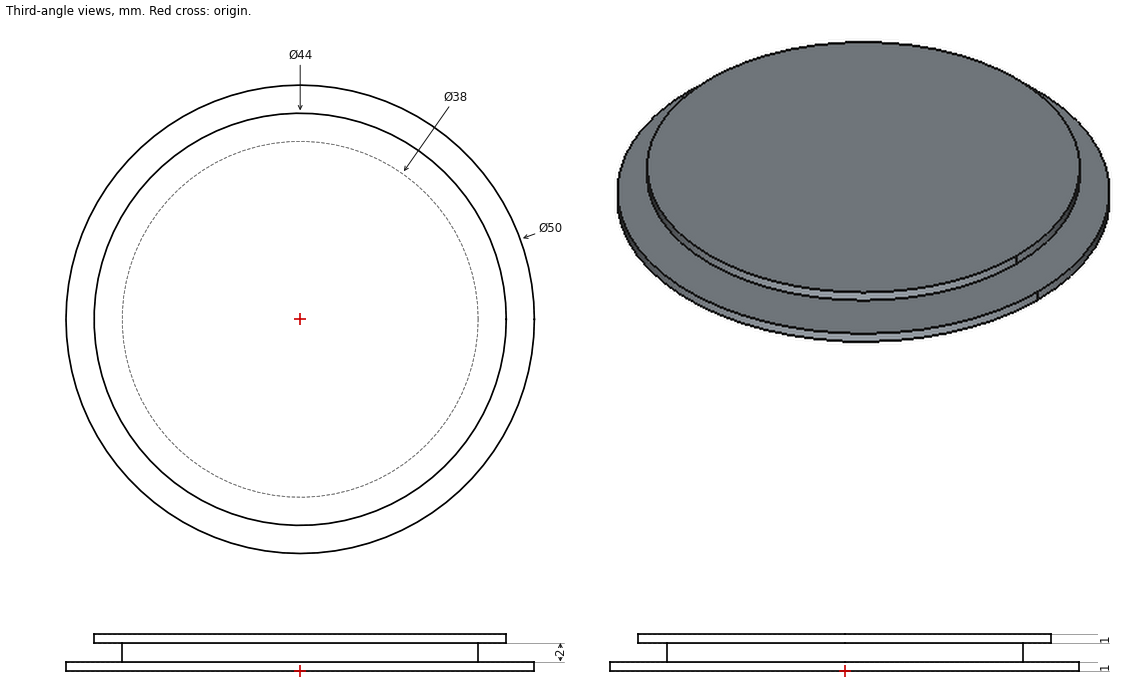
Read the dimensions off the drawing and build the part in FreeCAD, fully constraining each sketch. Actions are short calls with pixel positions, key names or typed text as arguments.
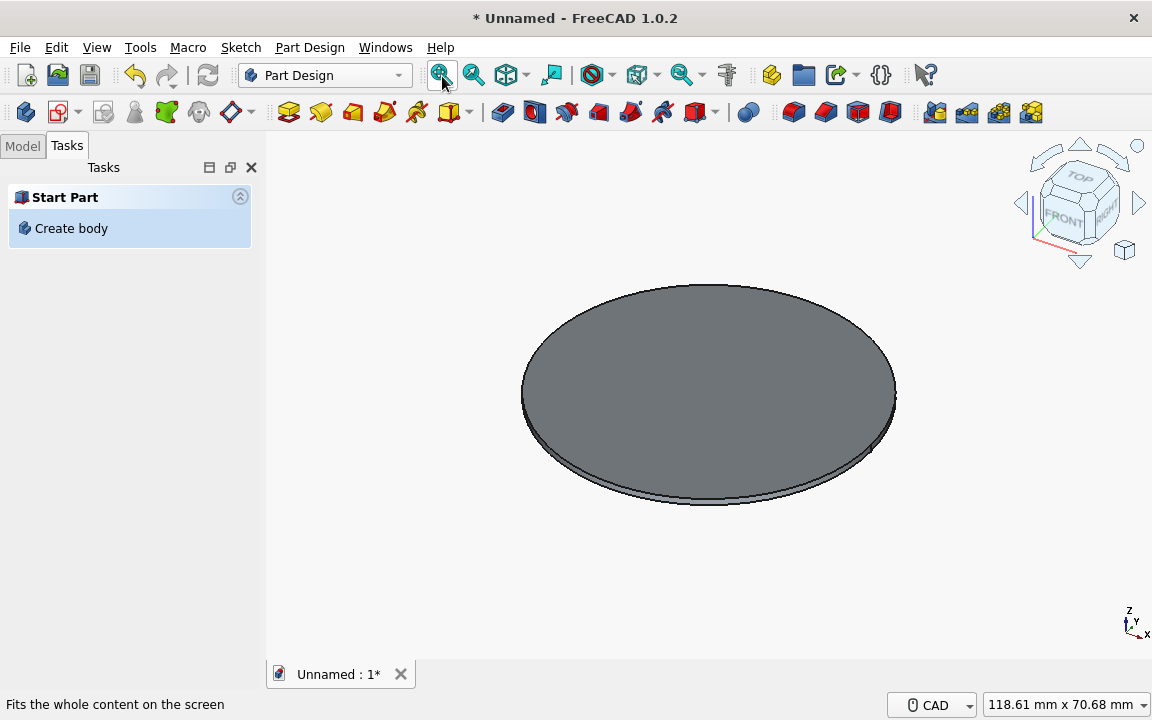
click(709, 391)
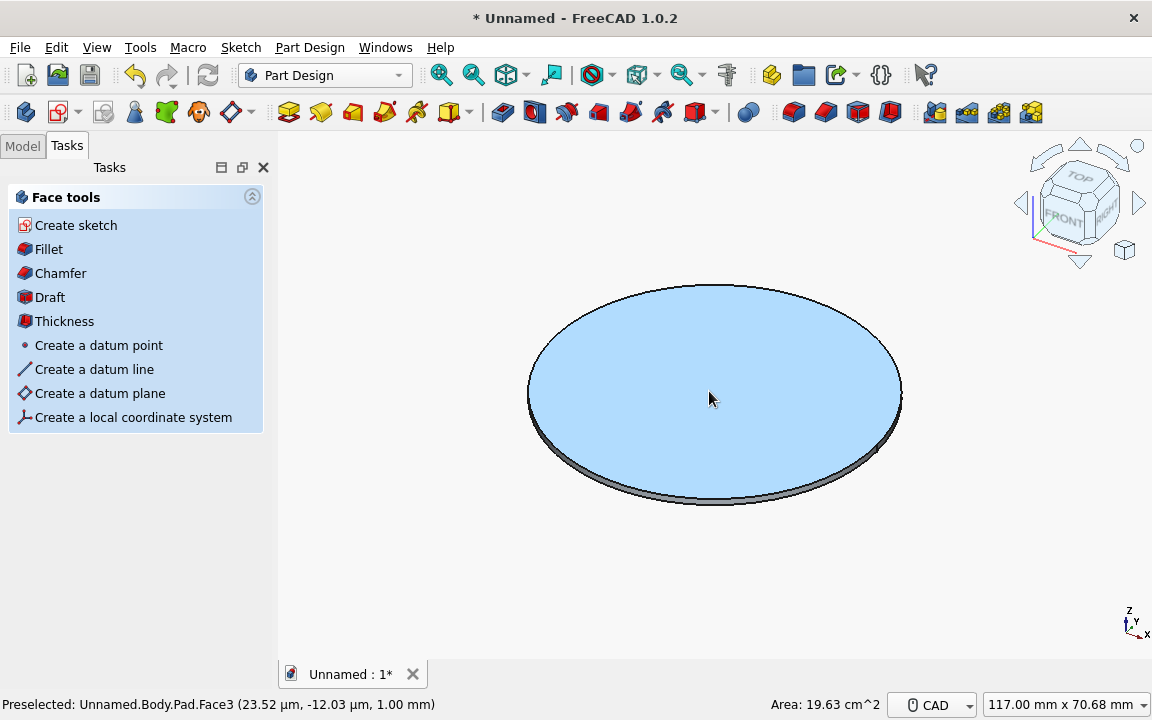
click(58, 112)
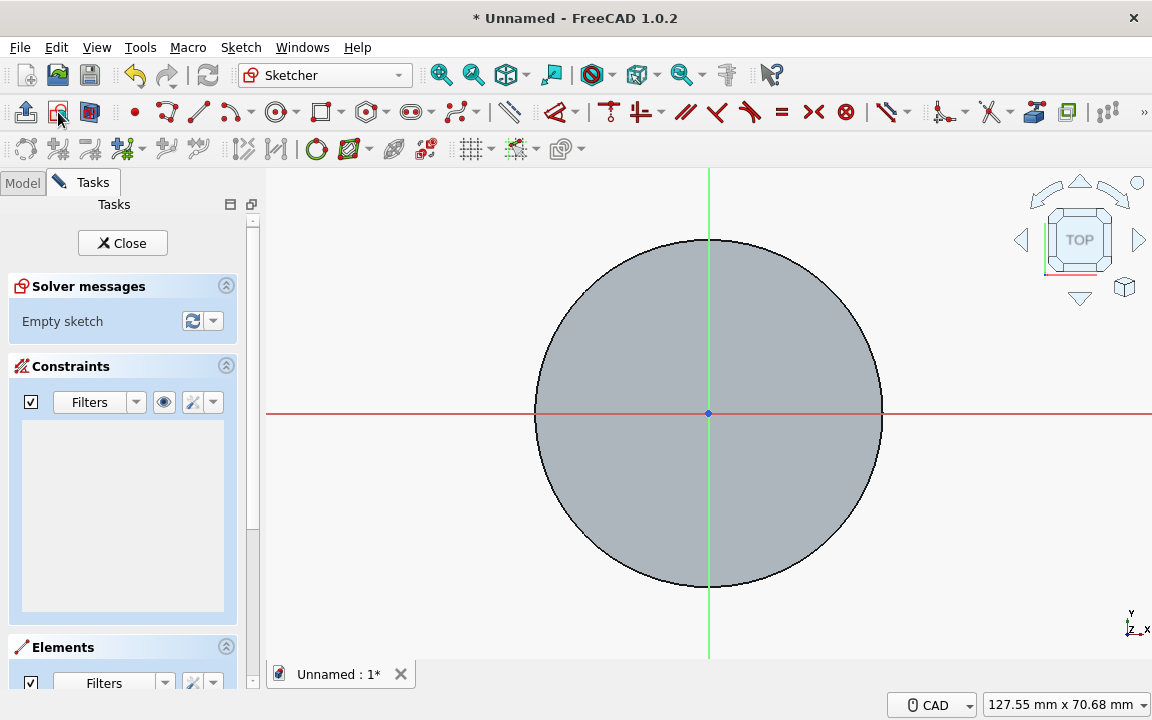
click(276, 112)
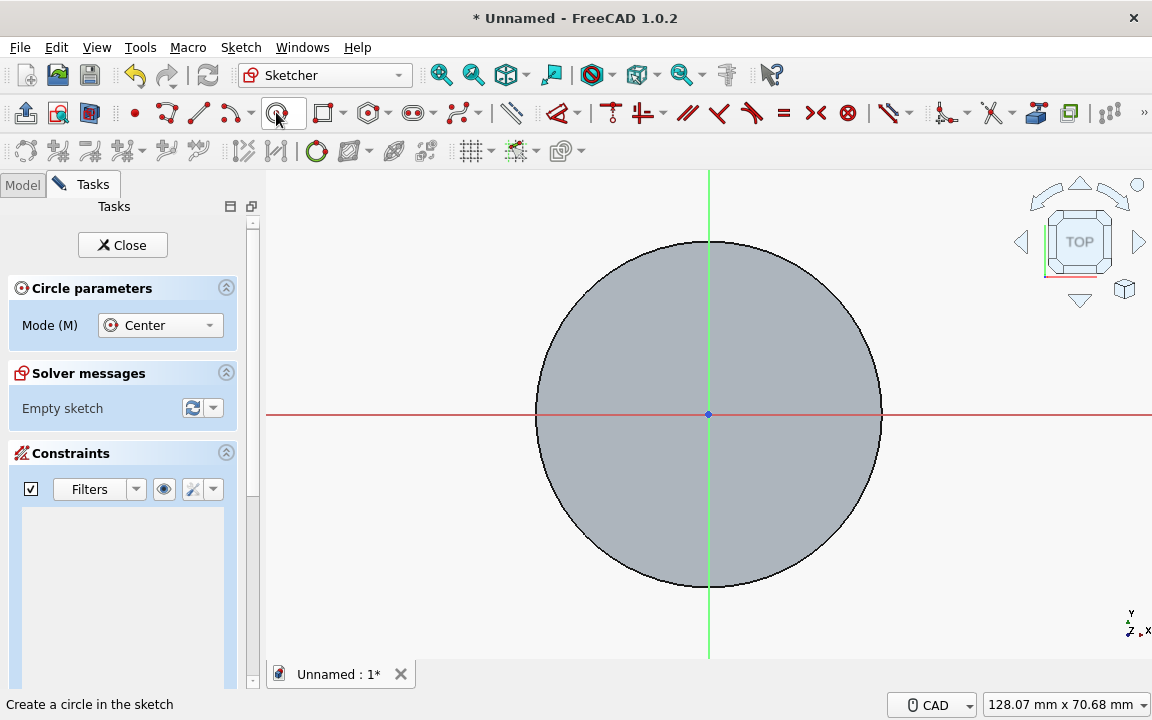
click(709, 414)
move(802, 322)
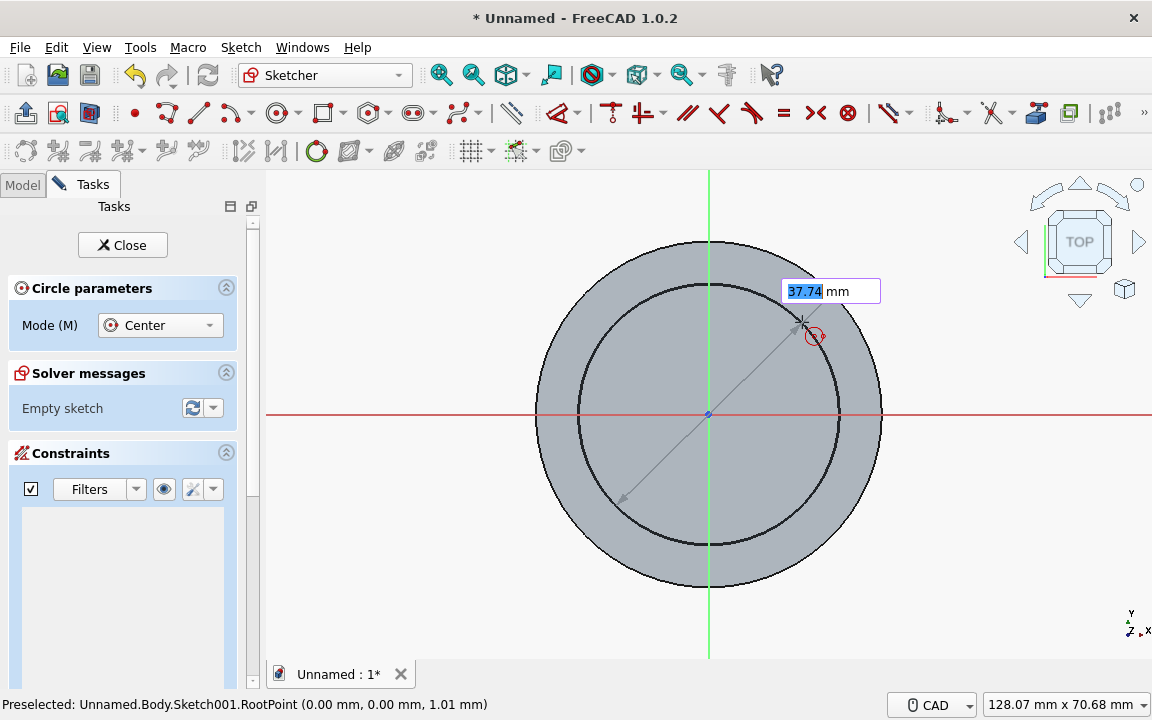
text(38)
key(Return)
key(Escape)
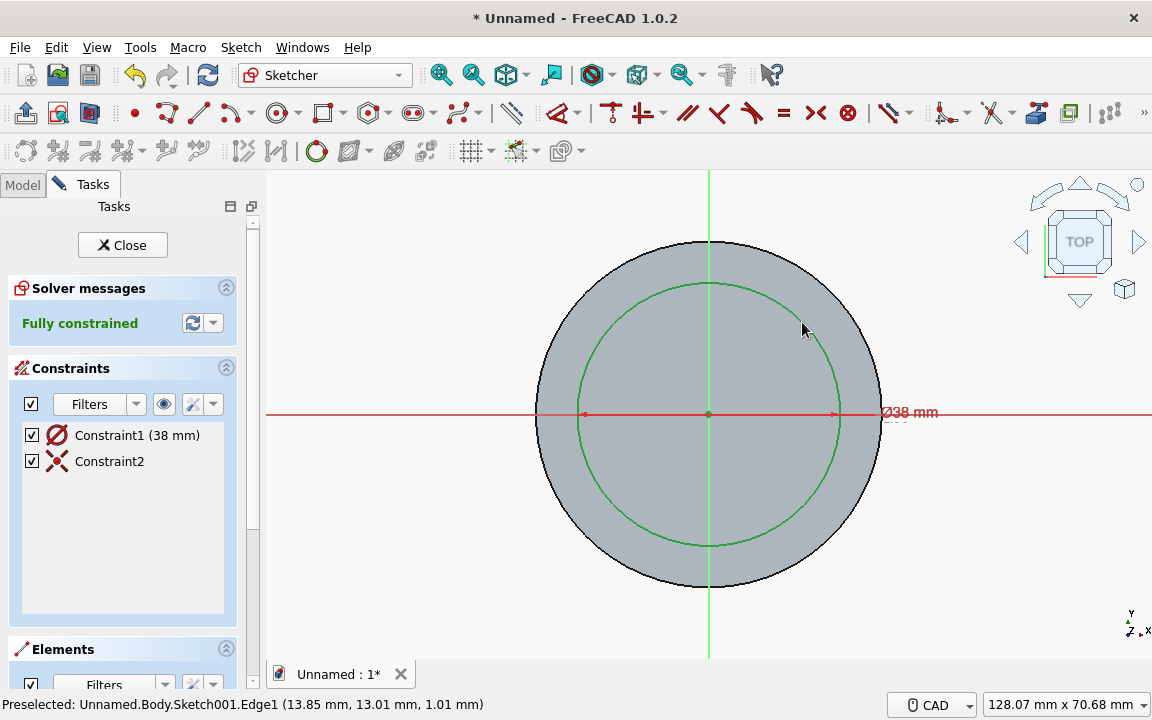
click(123, 245)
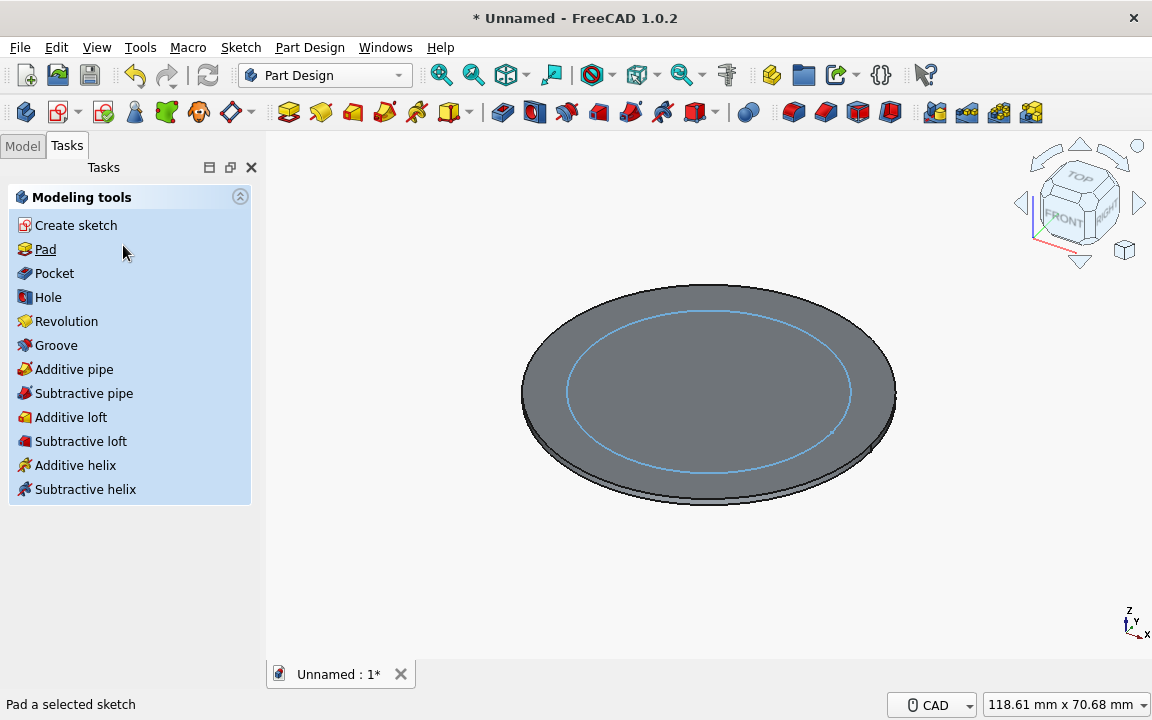
click(290, 112)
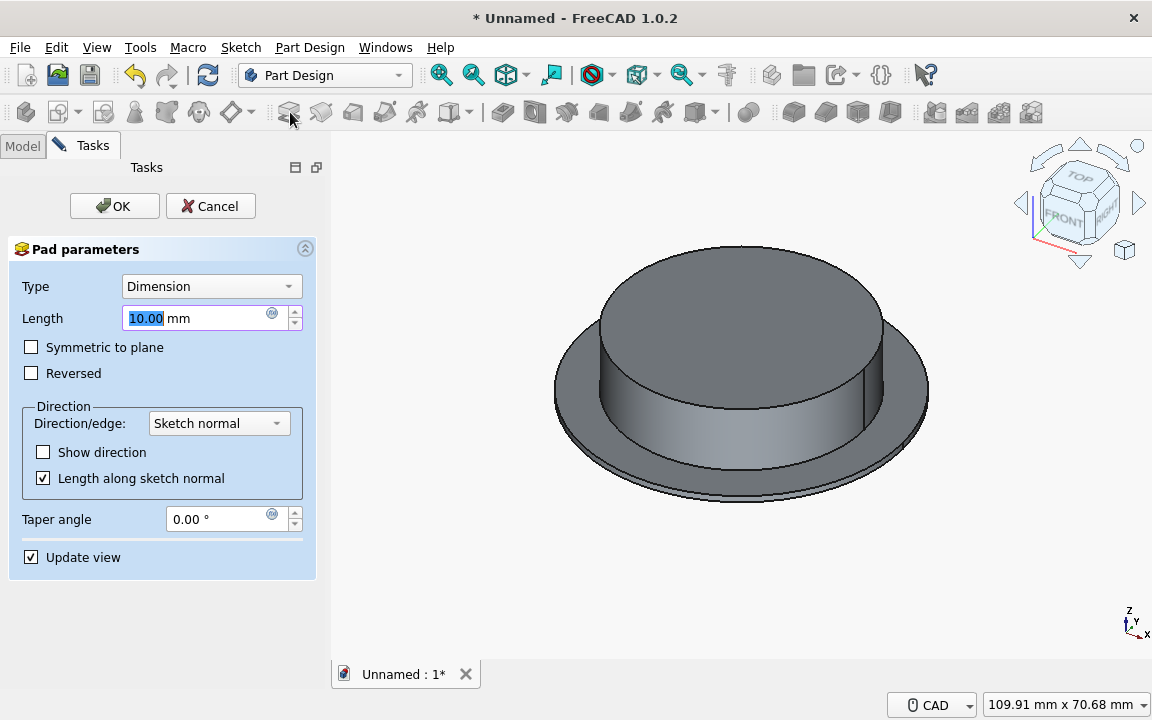
text(2)
key(Tab)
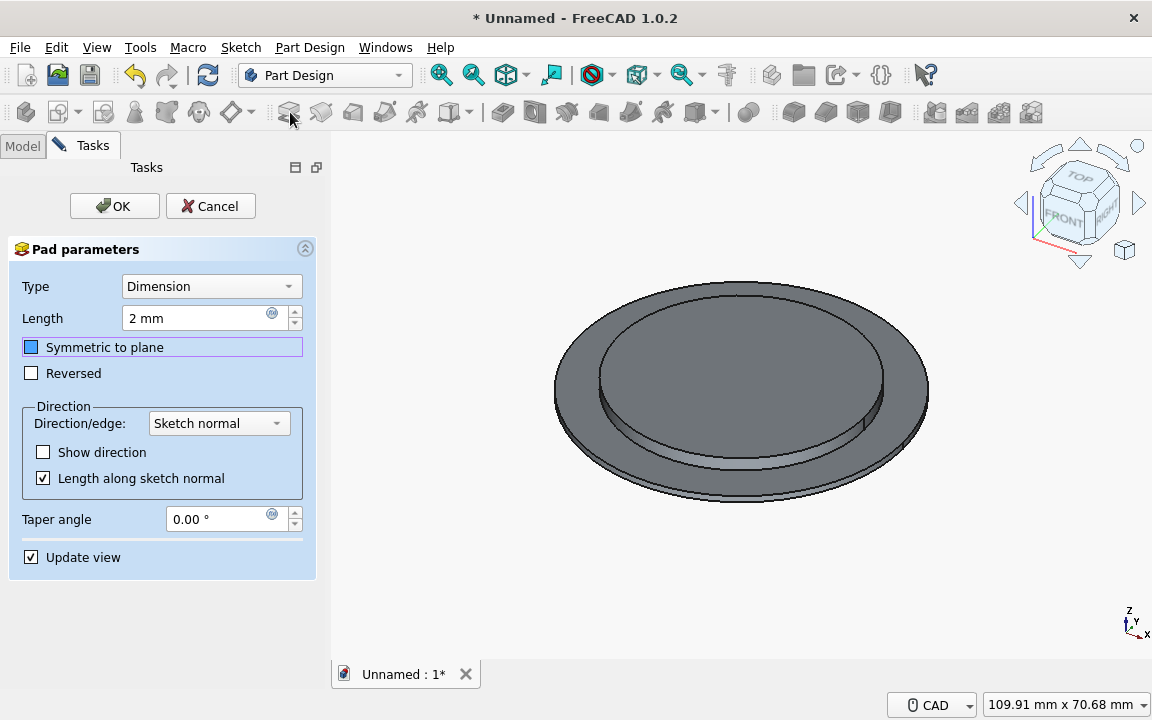
click(115, 206)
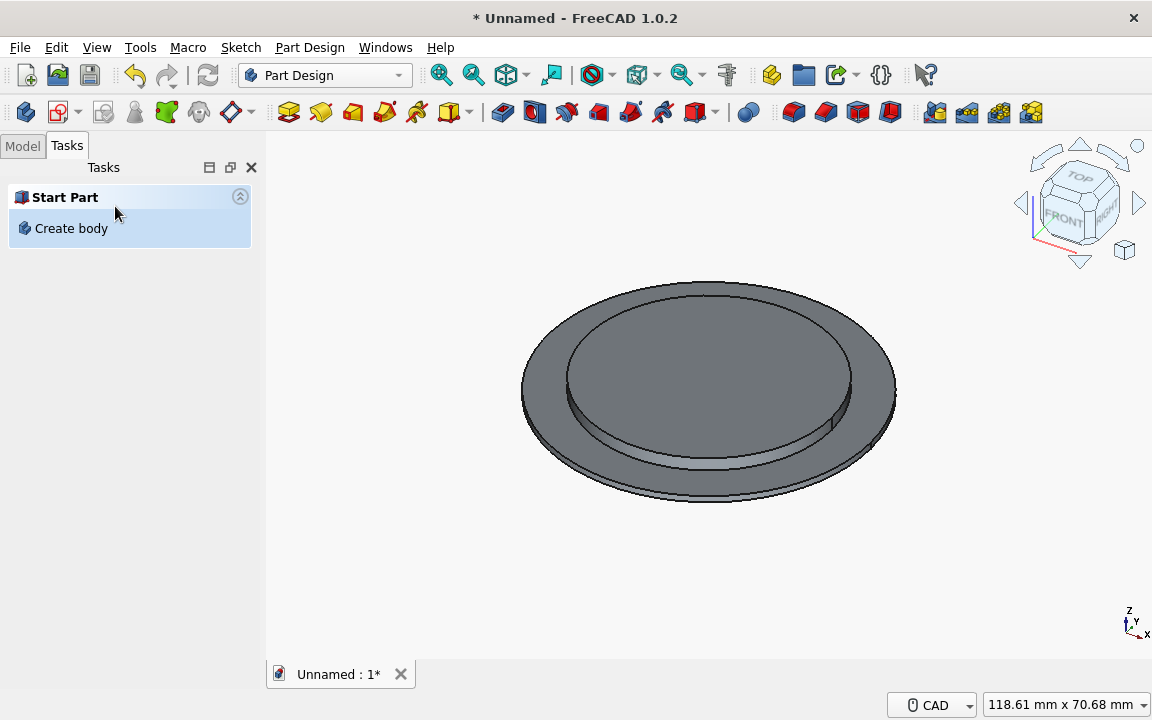
click(709, 376)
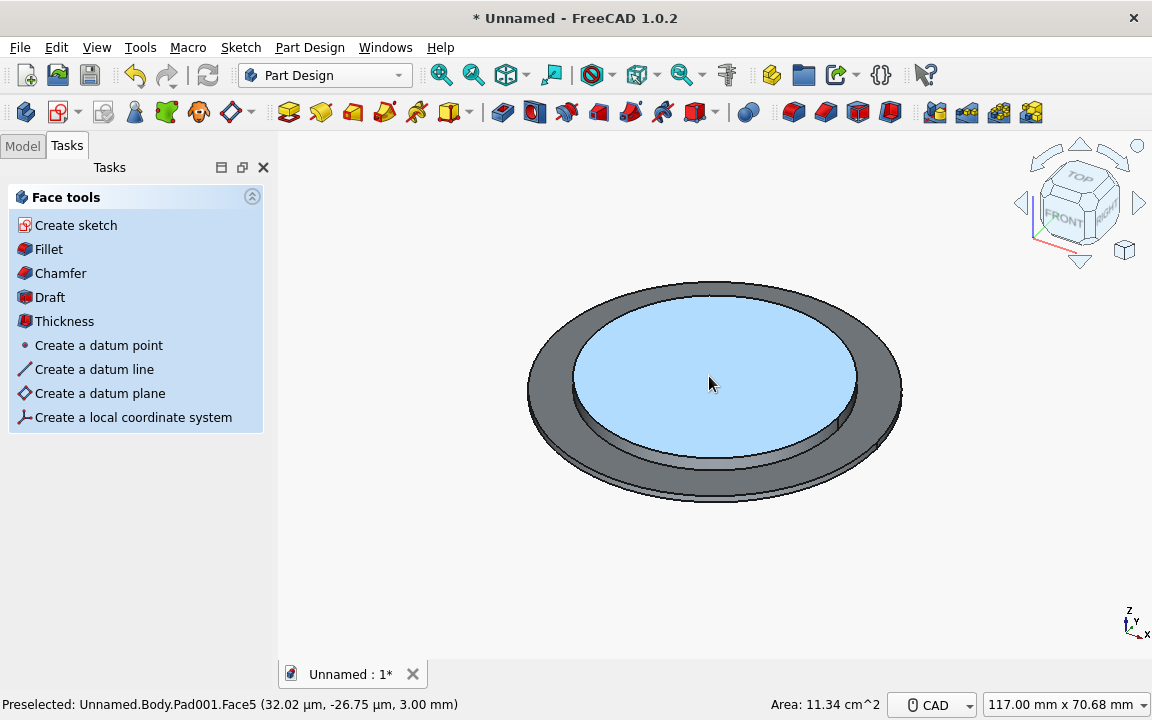
click(58, 112)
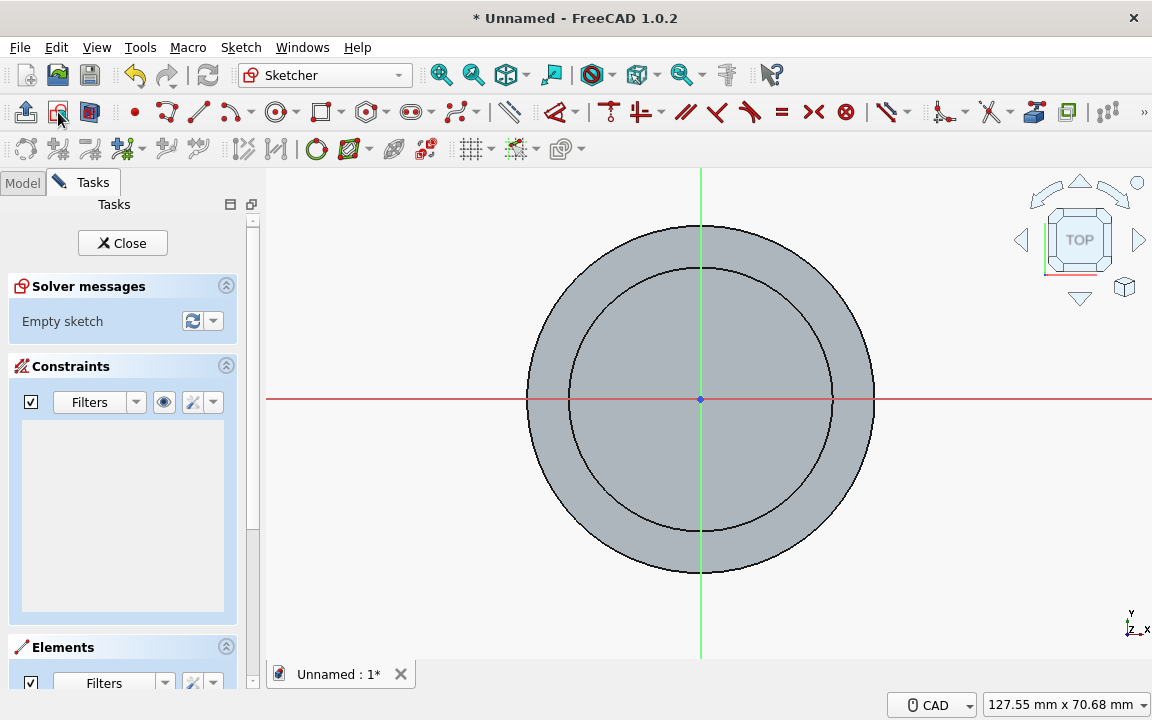
click(276, 112)